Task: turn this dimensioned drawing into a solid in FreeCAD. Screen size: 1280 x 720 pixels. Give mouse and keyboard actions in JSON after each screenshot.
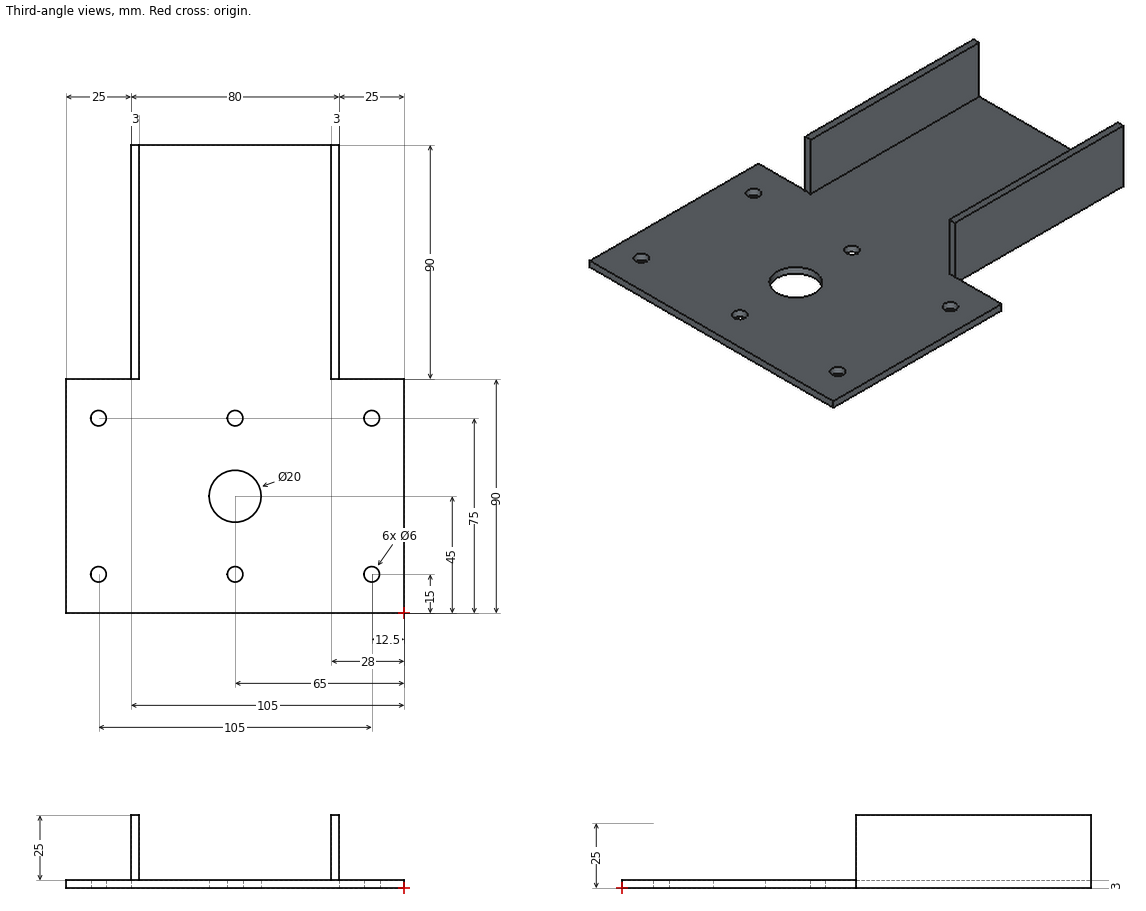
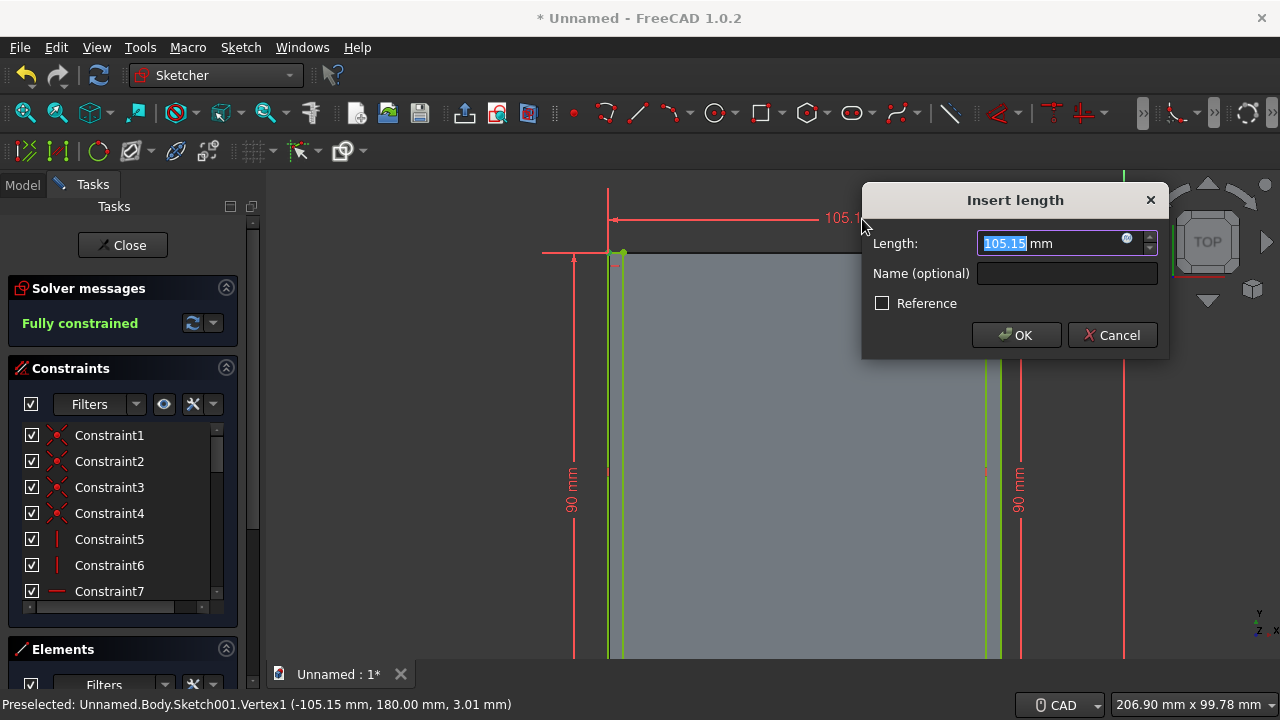
{"action": "type", "text": "105"}
{"action": "key", "text": "Return"}
{"action": "key", "text": "Escape"}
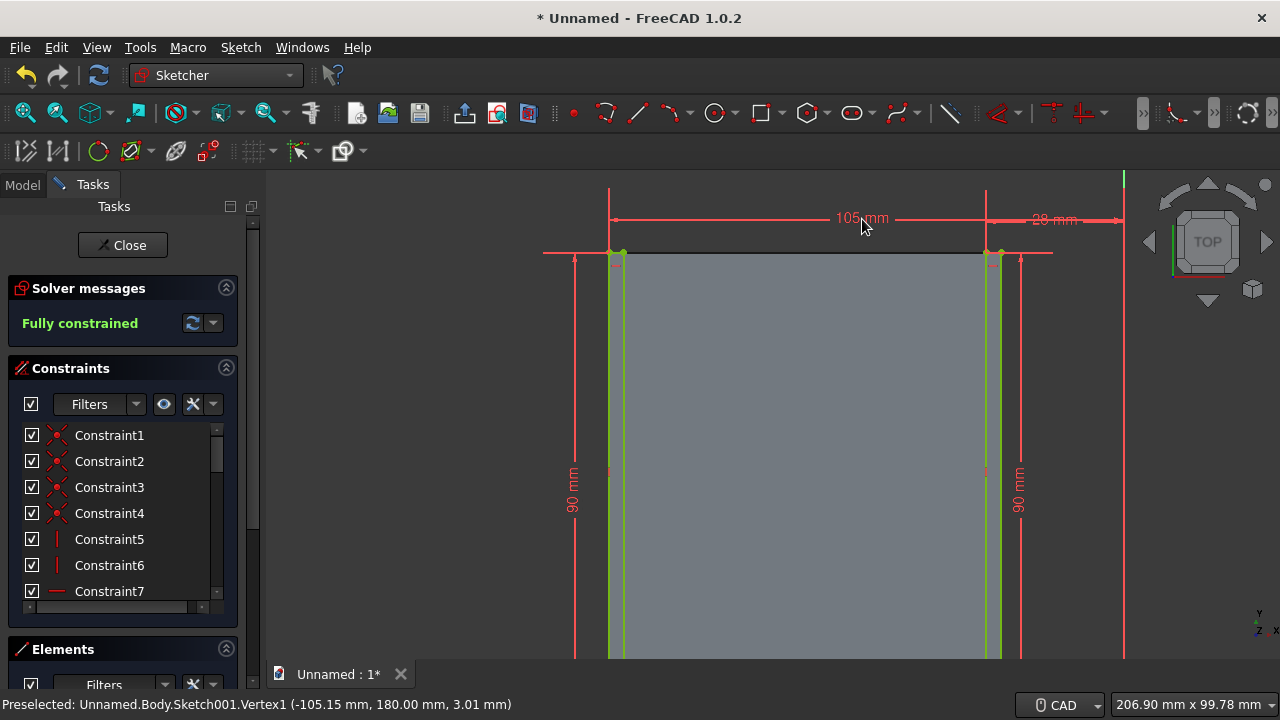
{"action": "left_click", "coordinate": [123, 245]}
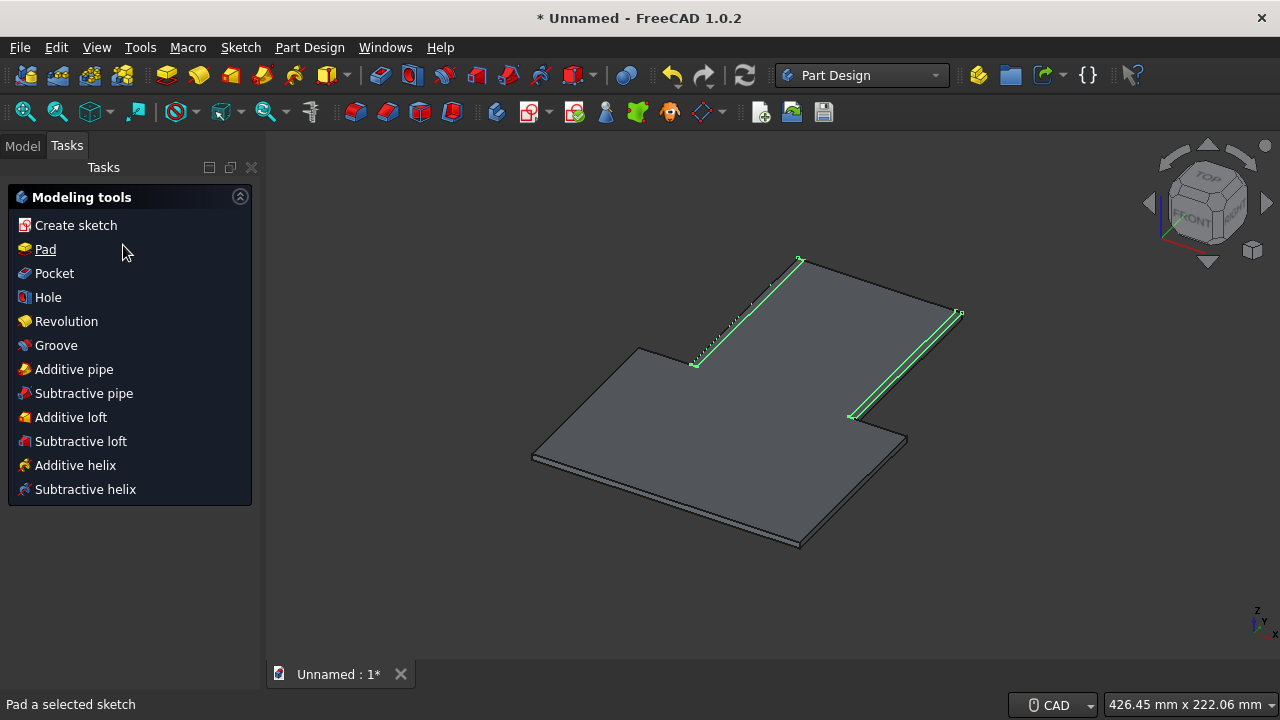
{"action": "left_click", "coordinate": [168, 76]}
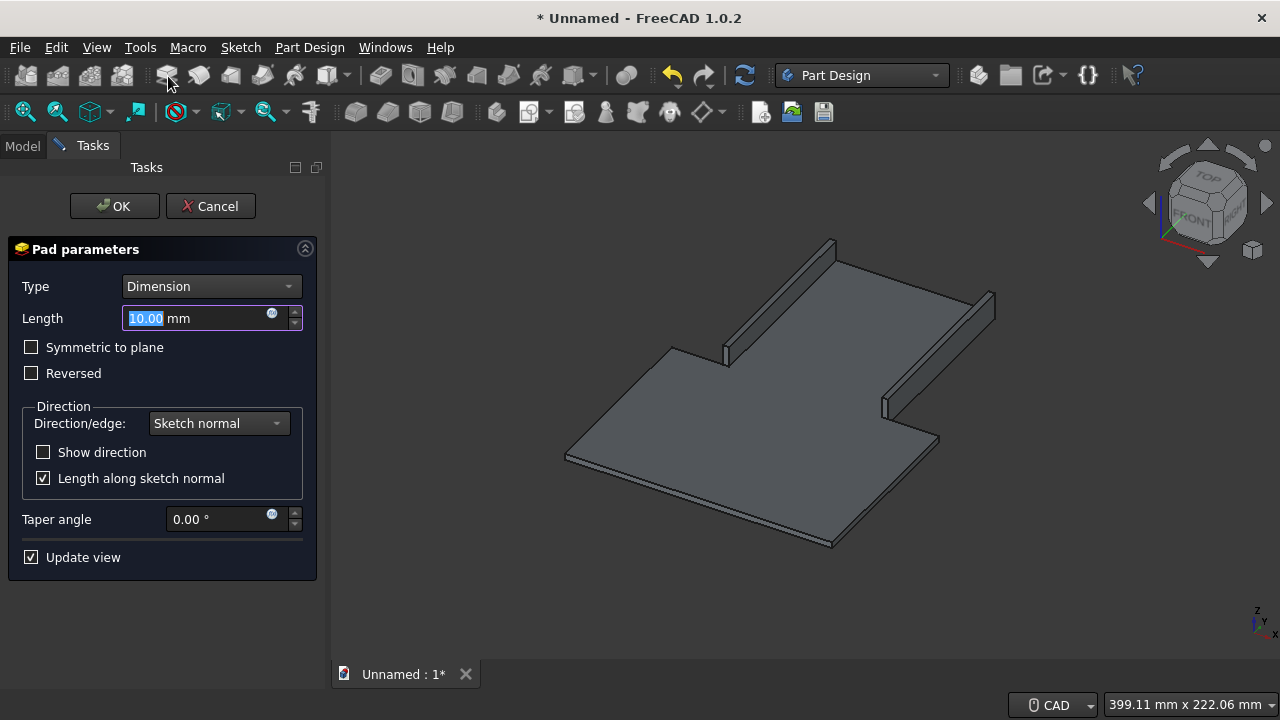
{"action": "type", "text": "25"}
{"action": "key", "text": "Tab"}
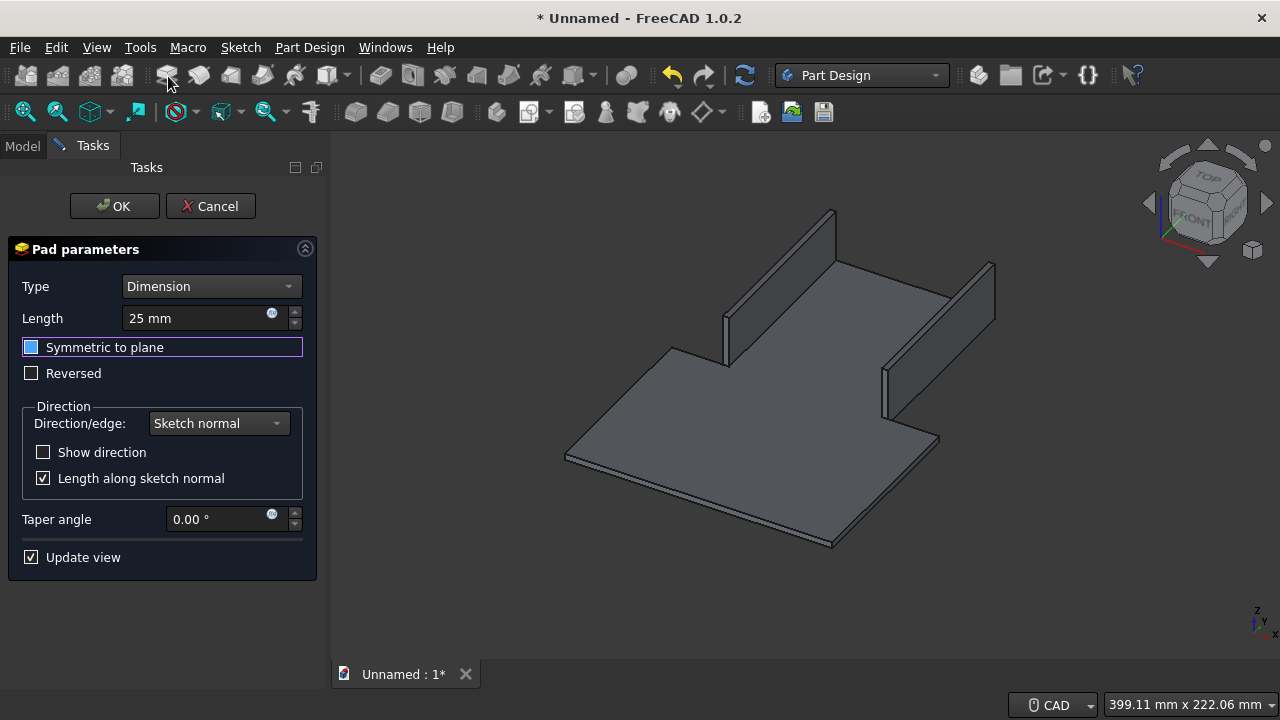
{"action": "left_click", "coordinate": [115, 206]}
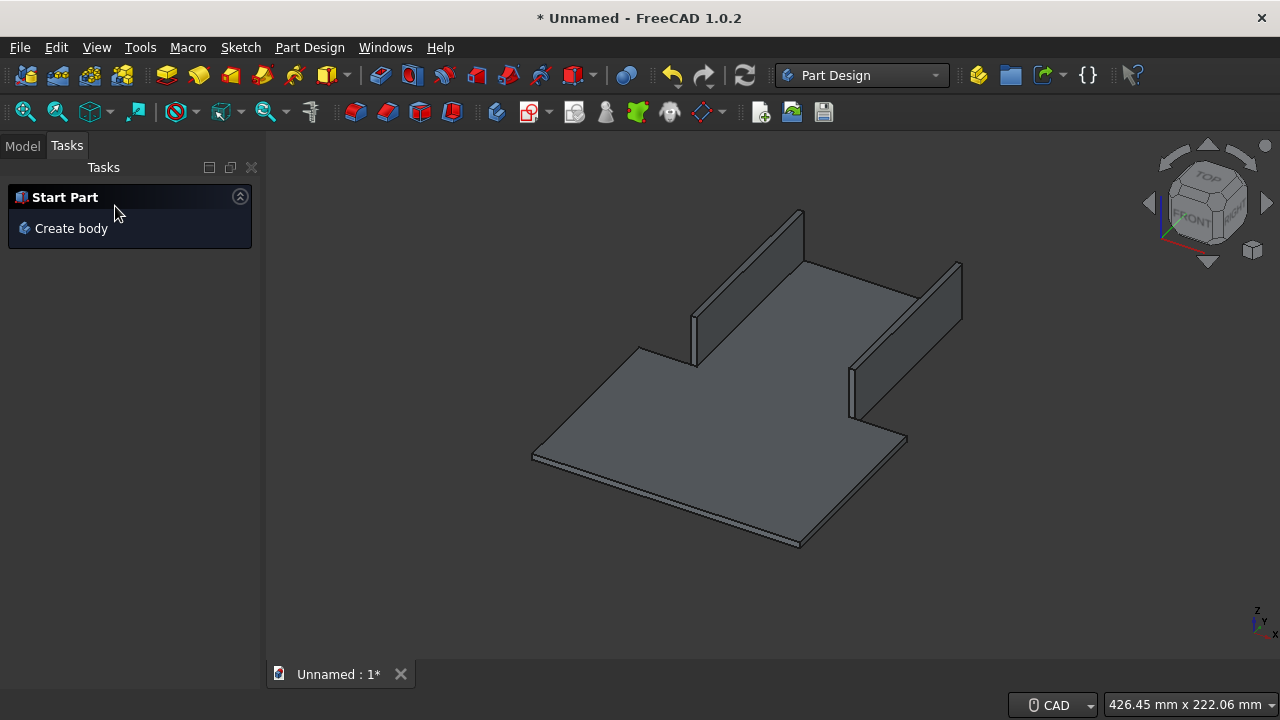
{"action": "left_click", "coordinate": [530, 112]}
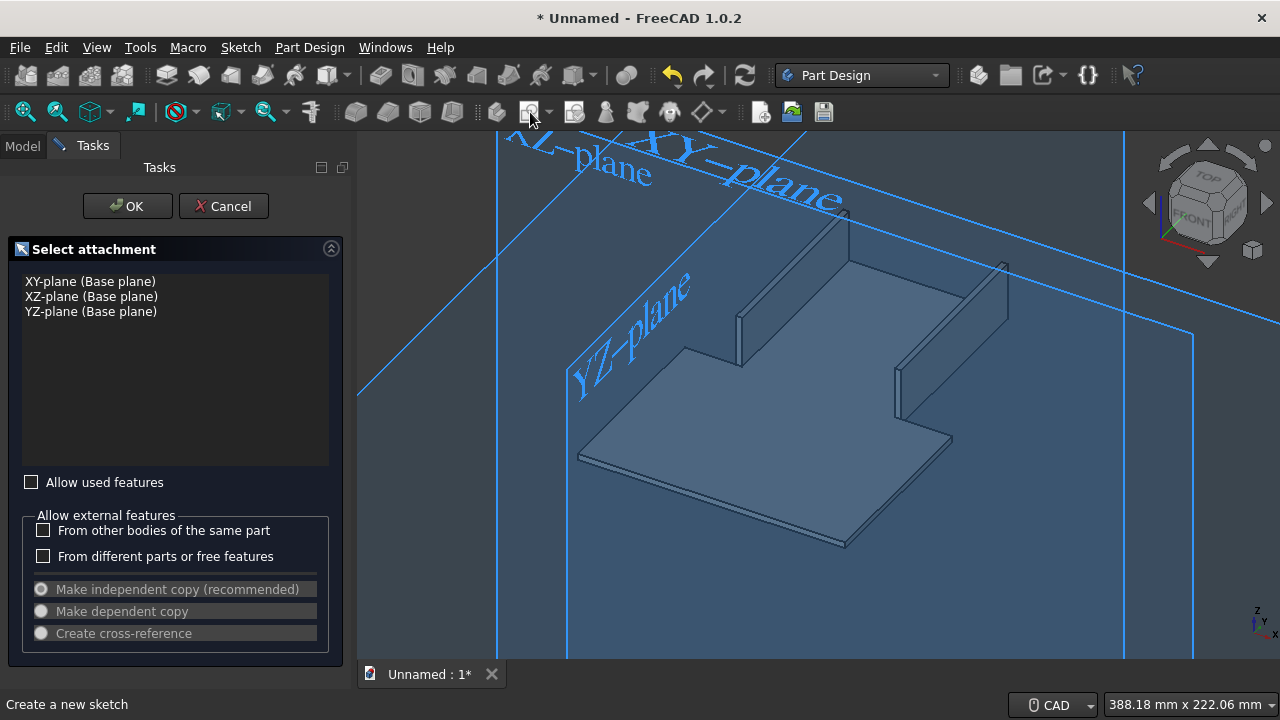
{"action": "left_click", "coordinate": [82, 282]}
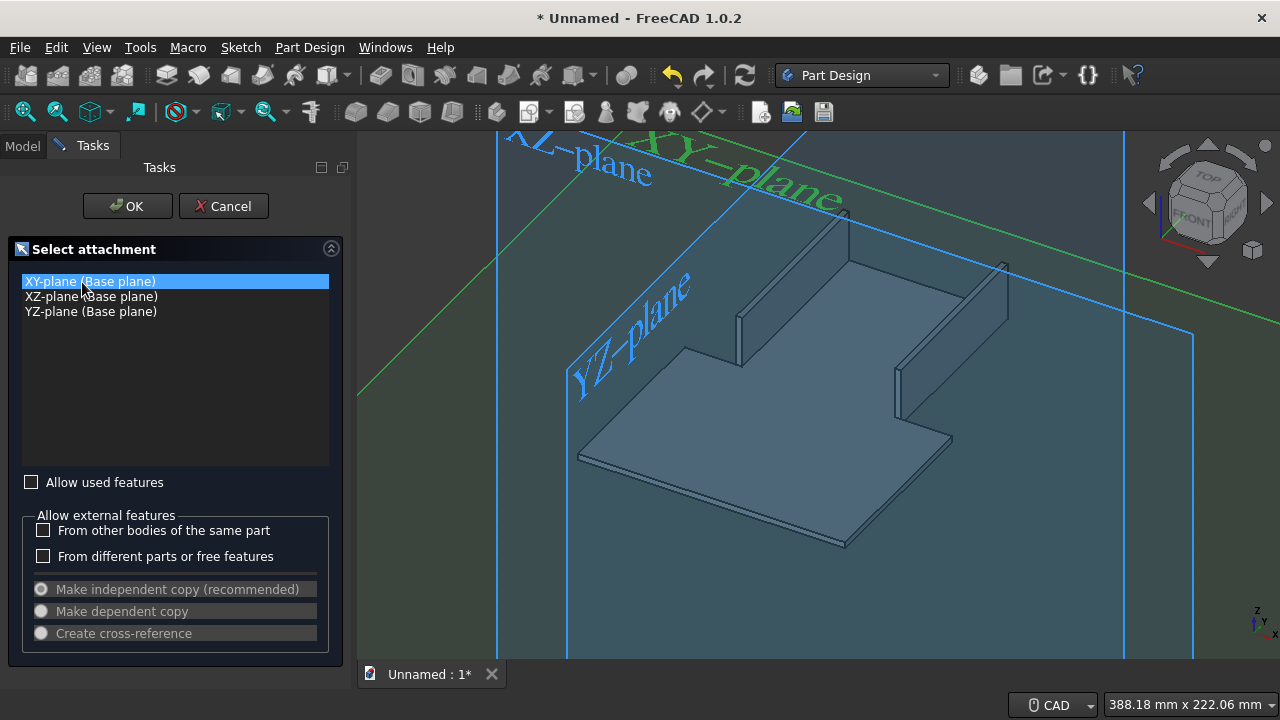
{"action": "left_click", "coordinate": [128, 206]}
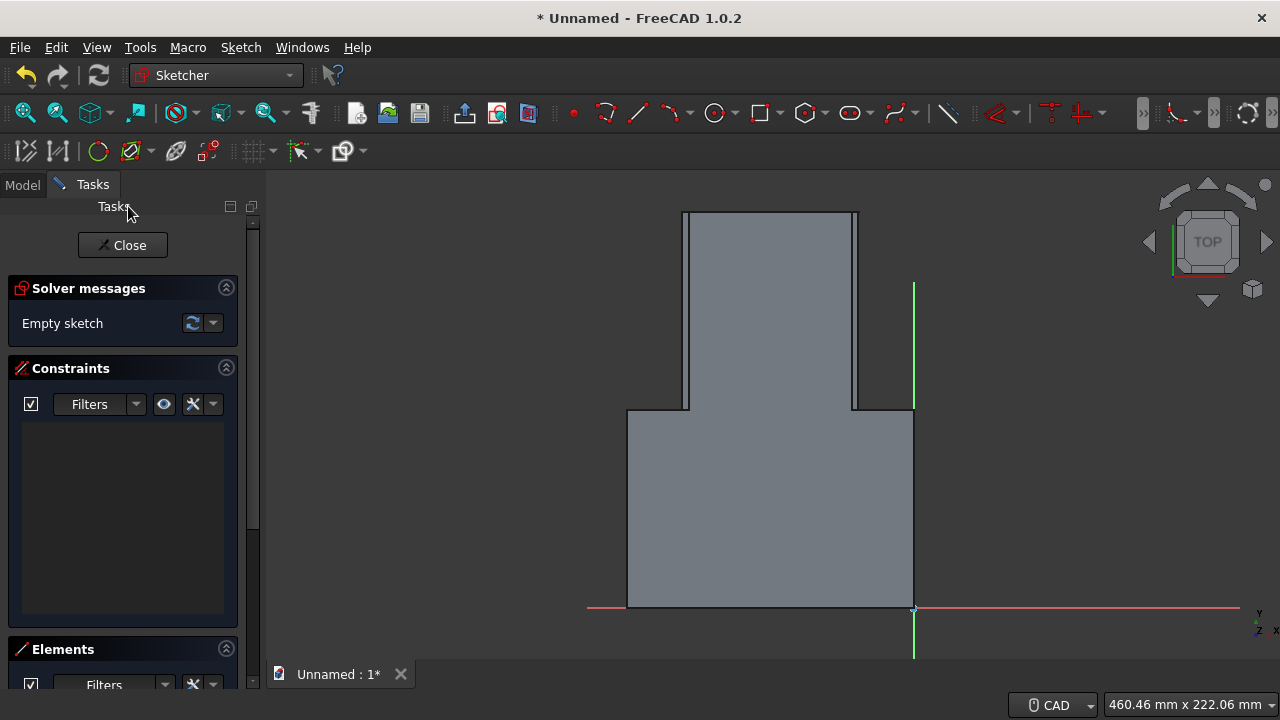
{"action": "left_click", "coordinate": [530, 114]}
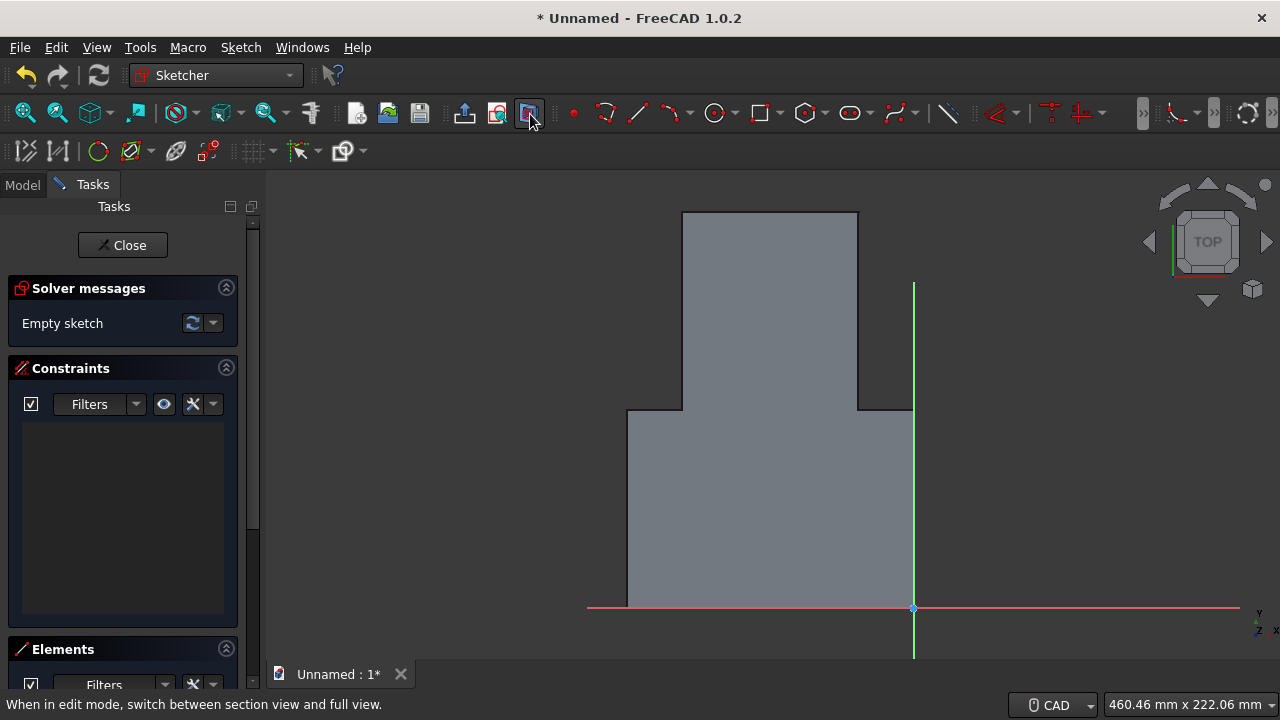
{"action": "scroll", "coordinate": [874, 631], "scroll_direction": "up", "scroll_amount": 3}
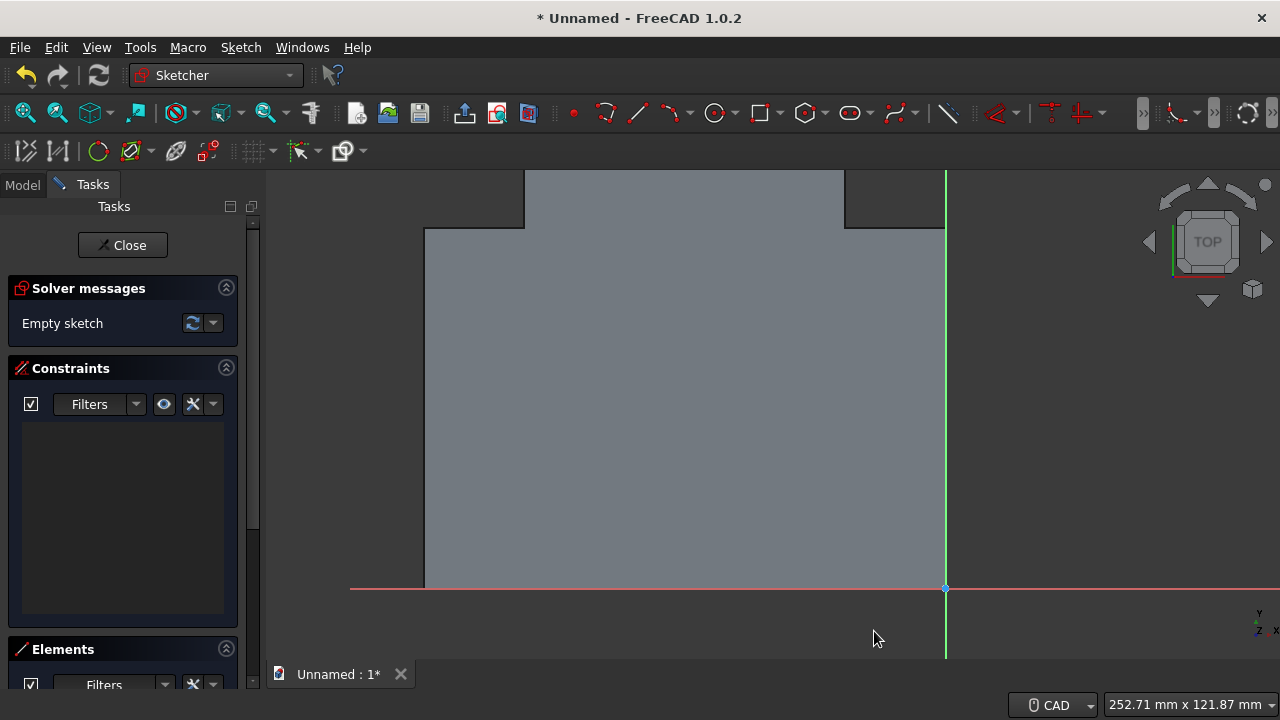
{"action": "key", "text": "g c"}